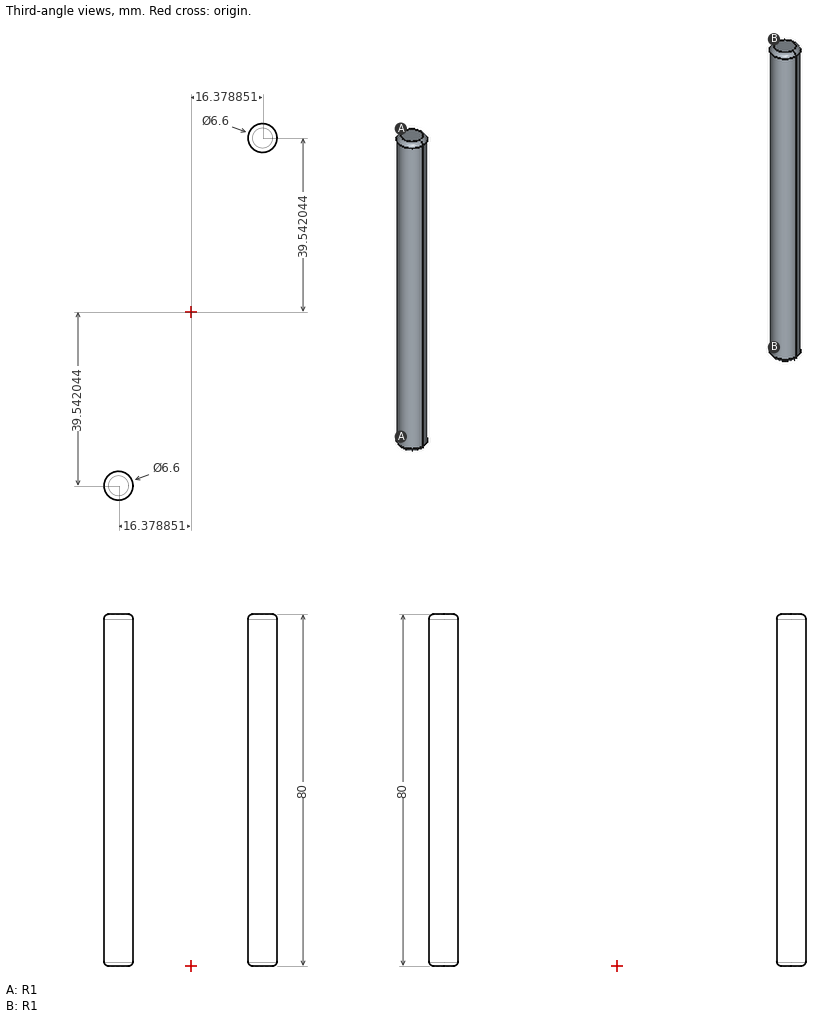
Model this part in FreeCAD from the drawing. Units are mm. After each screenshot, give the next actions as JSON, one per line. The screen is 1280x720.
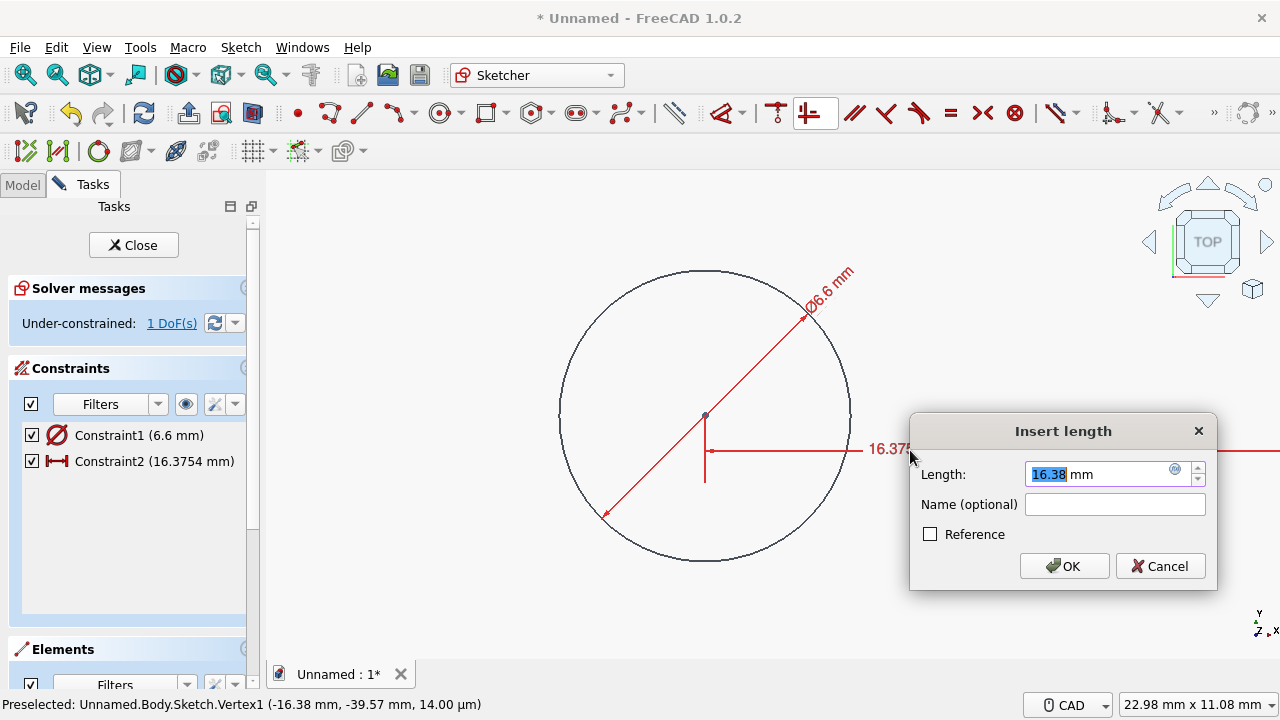
{"action": "type", "text": "16.378851"}
{"action": "key", "text": "Return"}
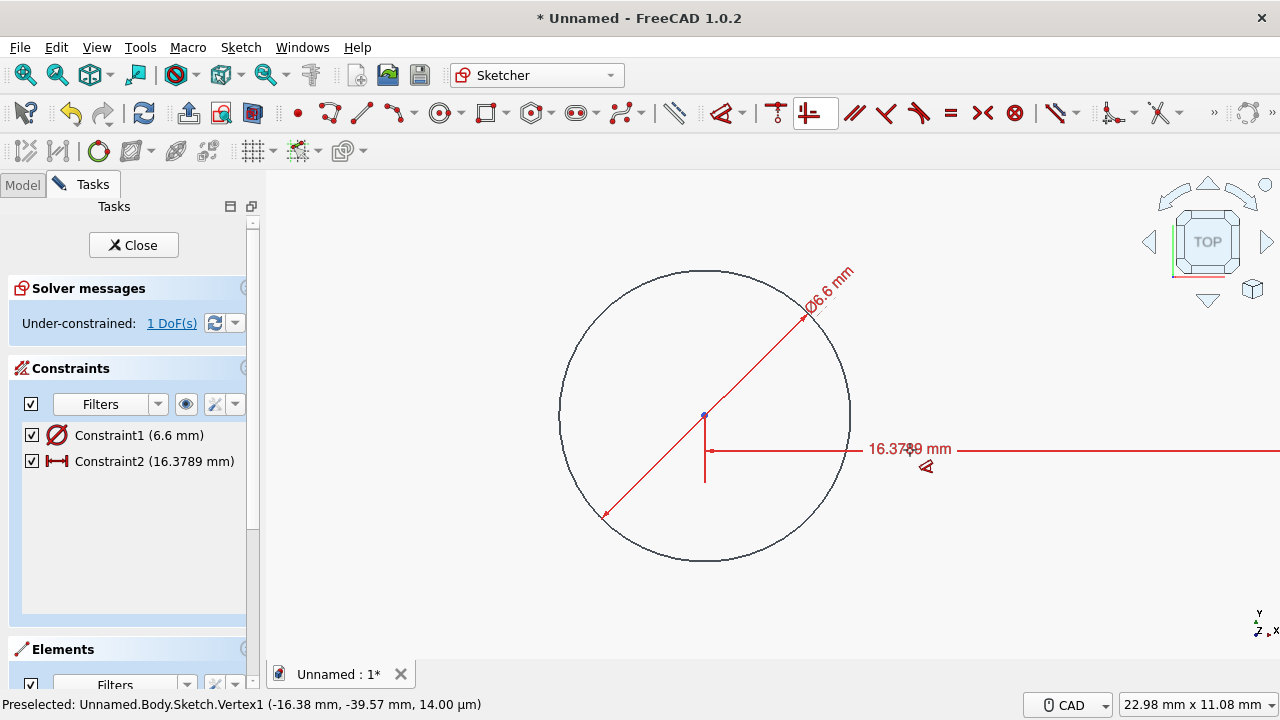
{"action": "left_click", "coordinate": [705, 416]}
{"action": "left_click", "coordinate": [671, 307]}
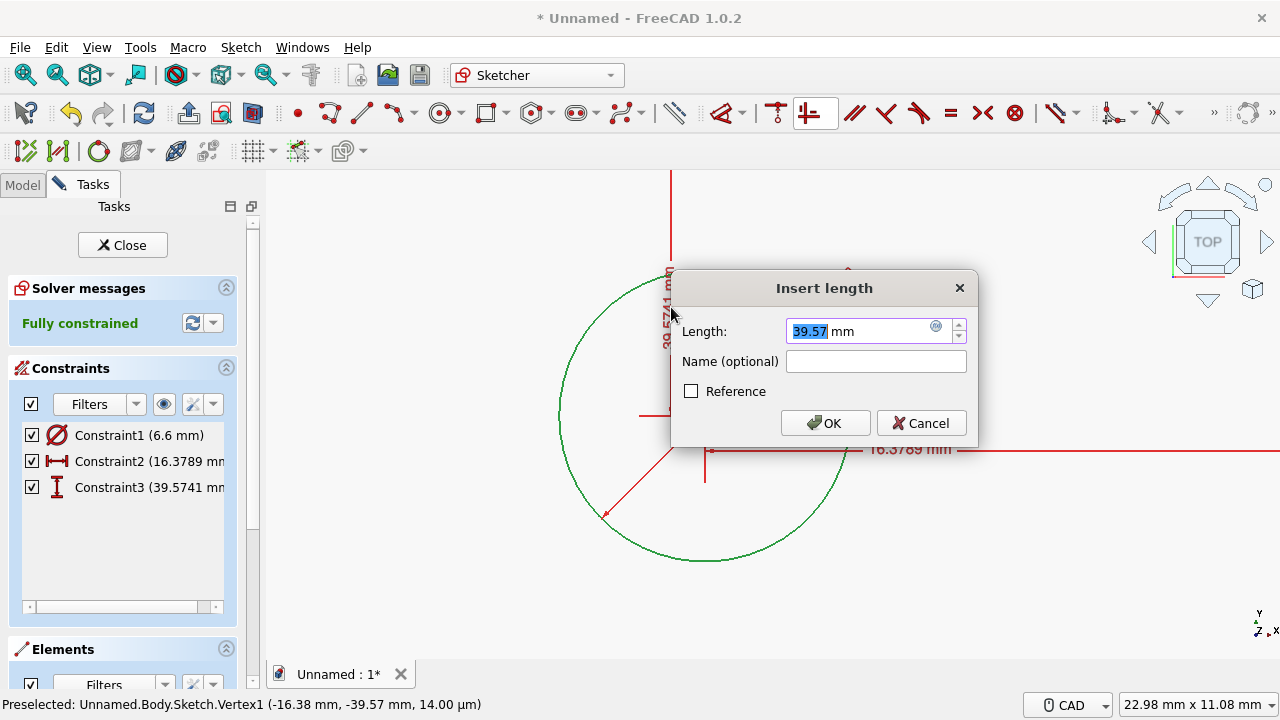
{"action": "type", "text": "39.542044"}
{"action": "key", "text": "Return"}
{"action": "key", "text": "Escape"}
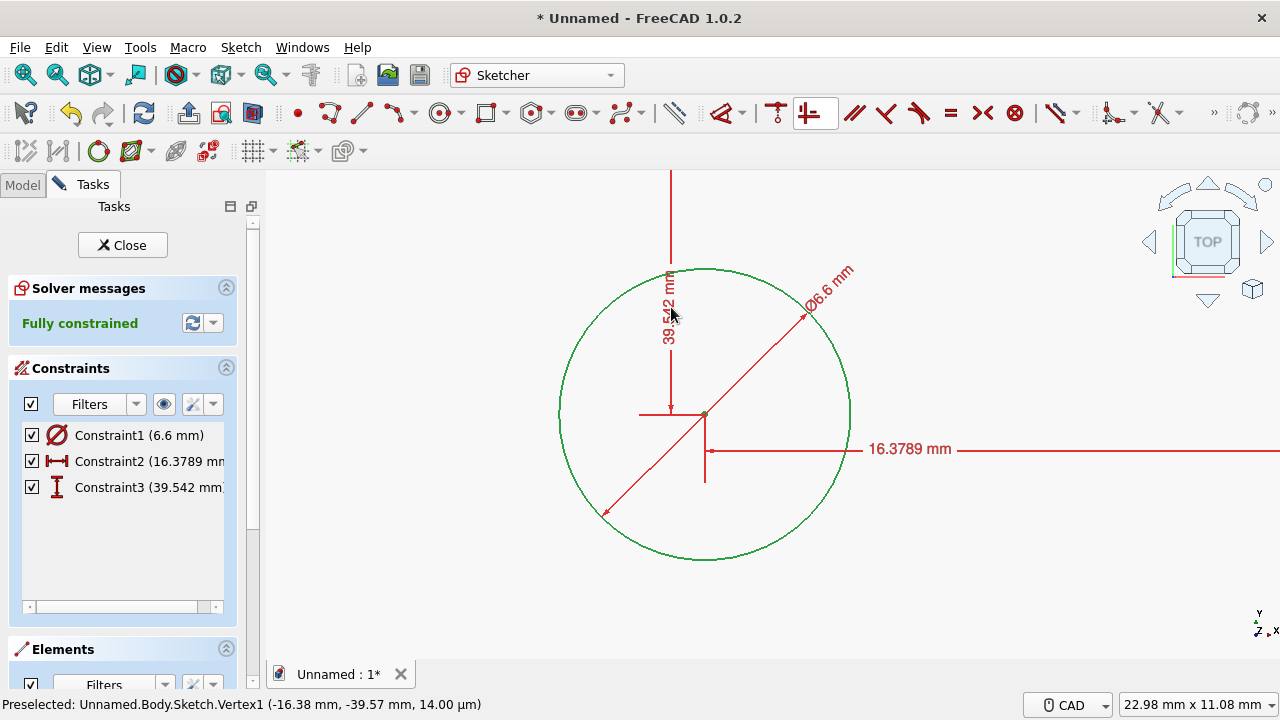
{"action": "left_click", "coordinate": [123, 245]}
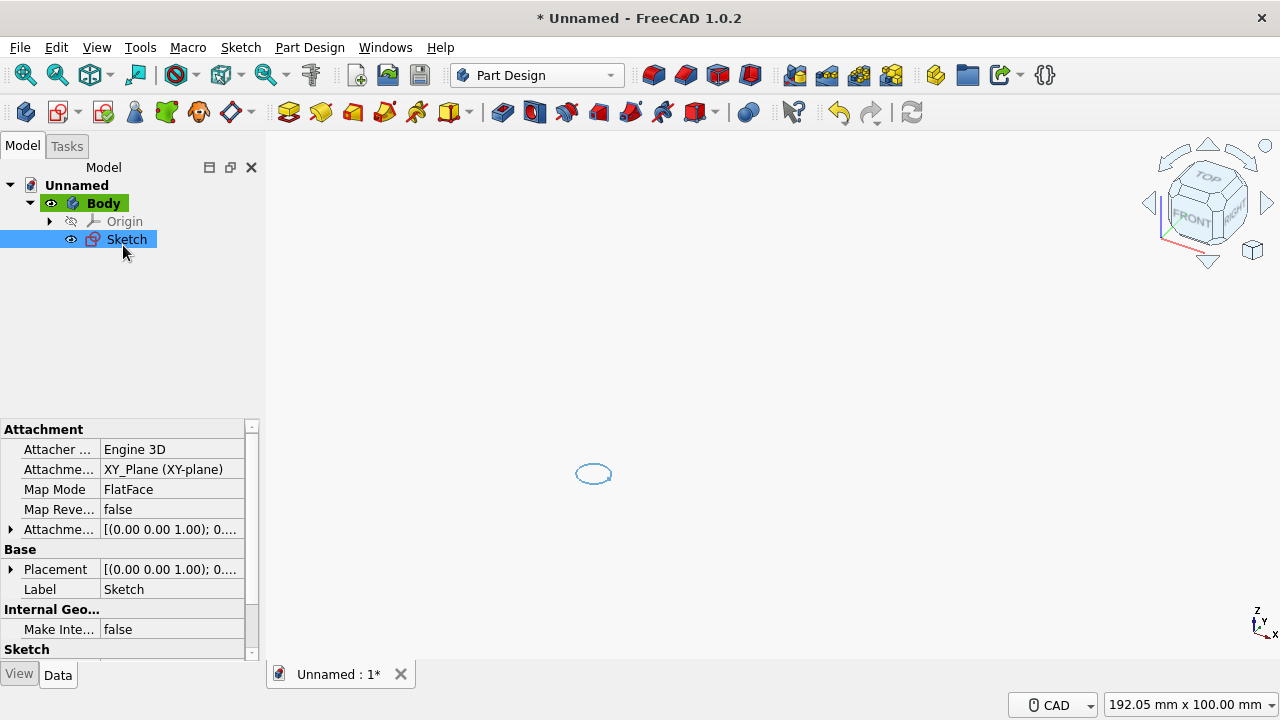
{"action": "left_click", "coordinate": [290, 112]}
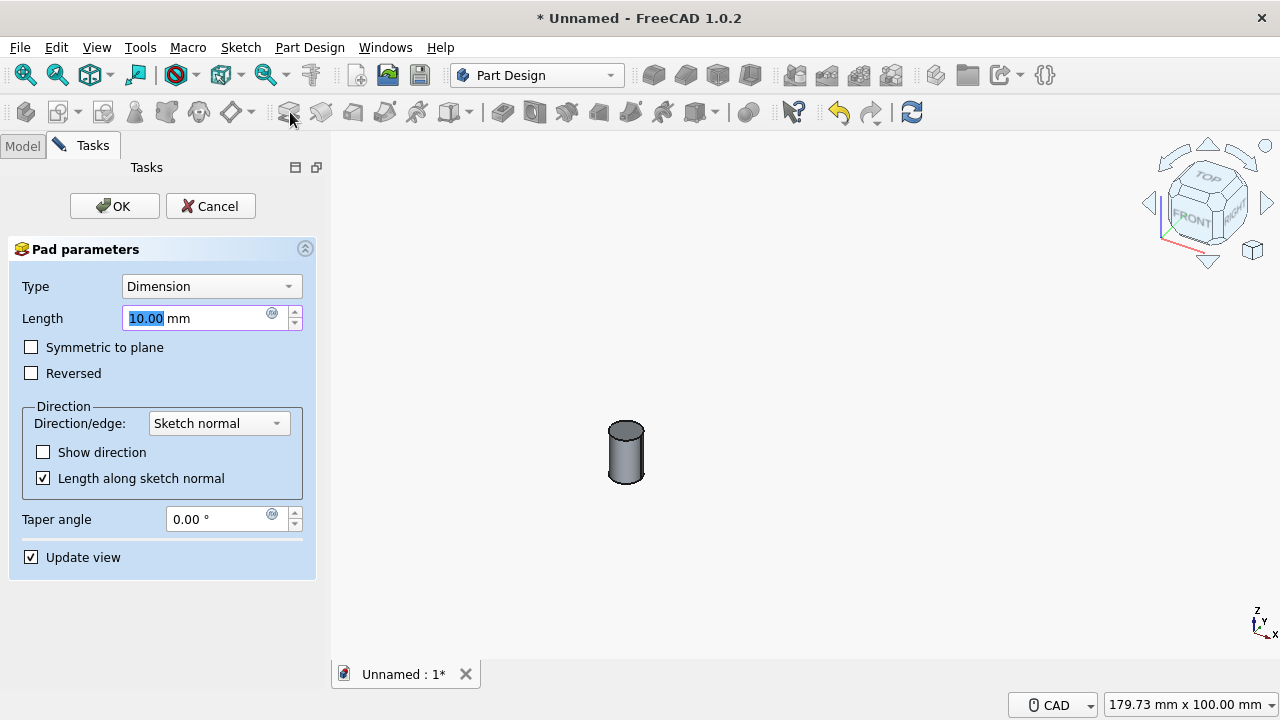
{"action": "type", "text": "80"}
{"action": "key", "text": "Tab"}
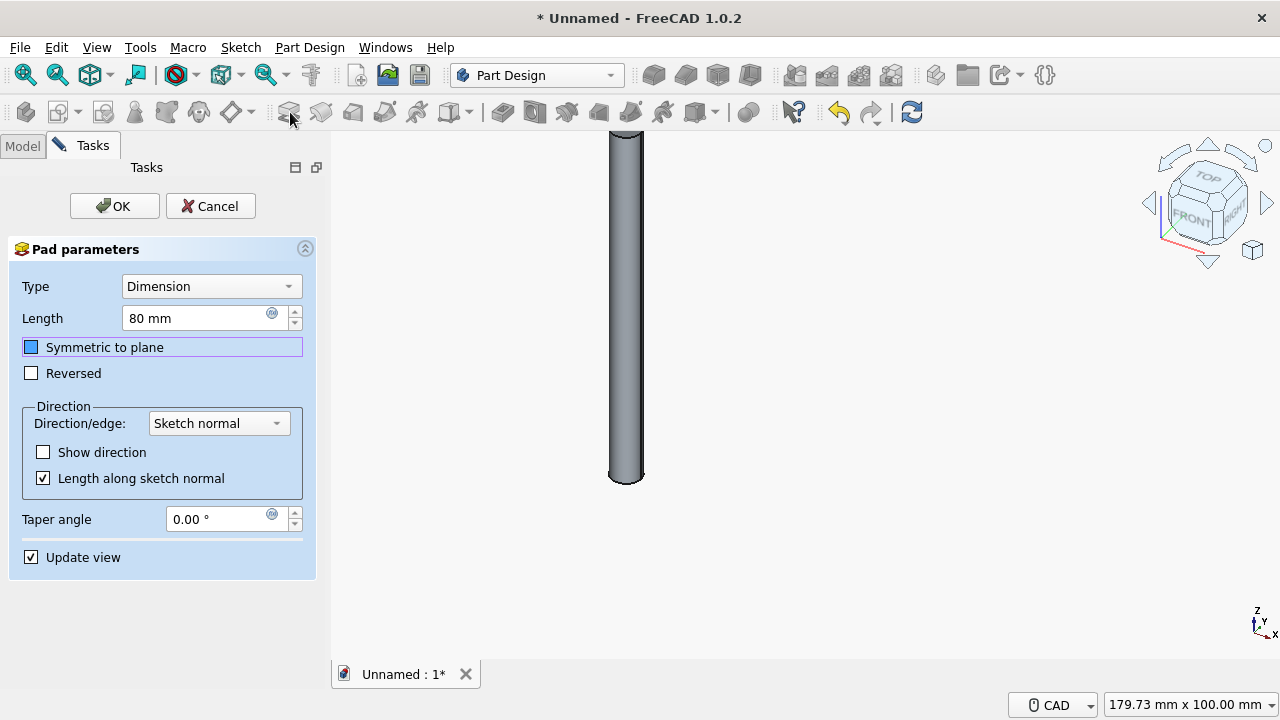
{"action": "left_click", "coordinate": [115, 206]}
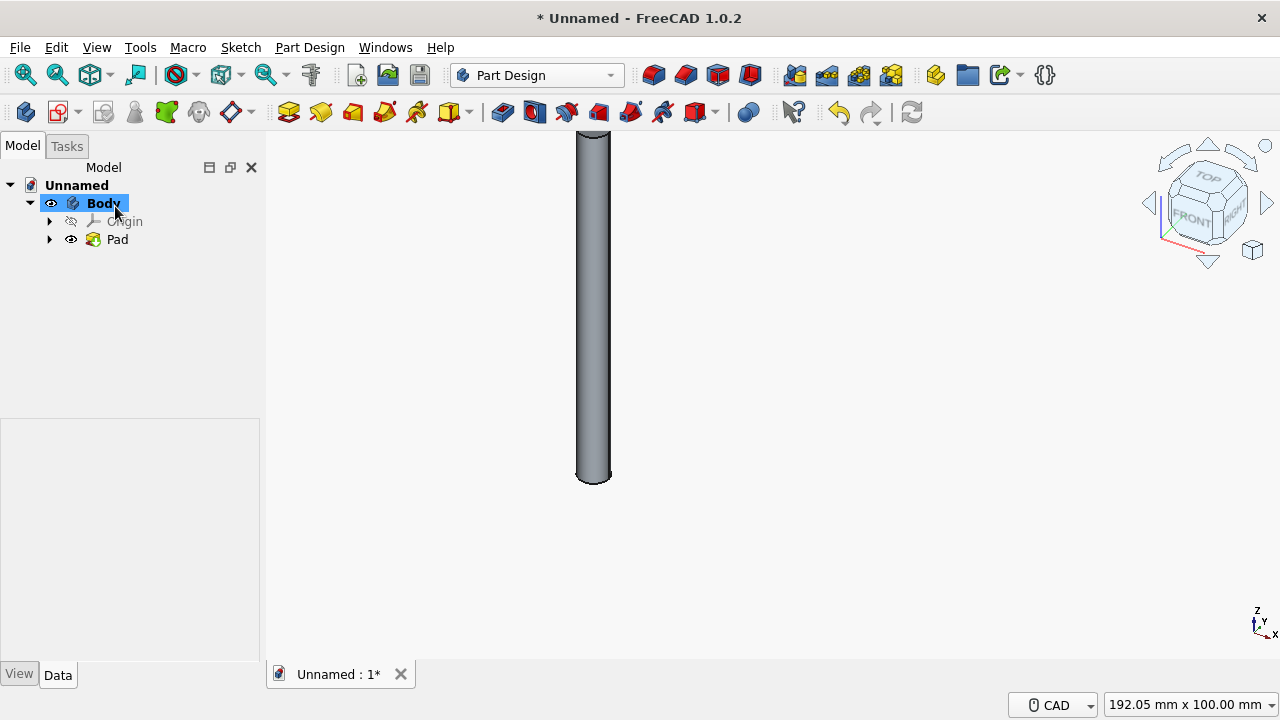
{"action": "left_click", "coordinate": [26, 76]}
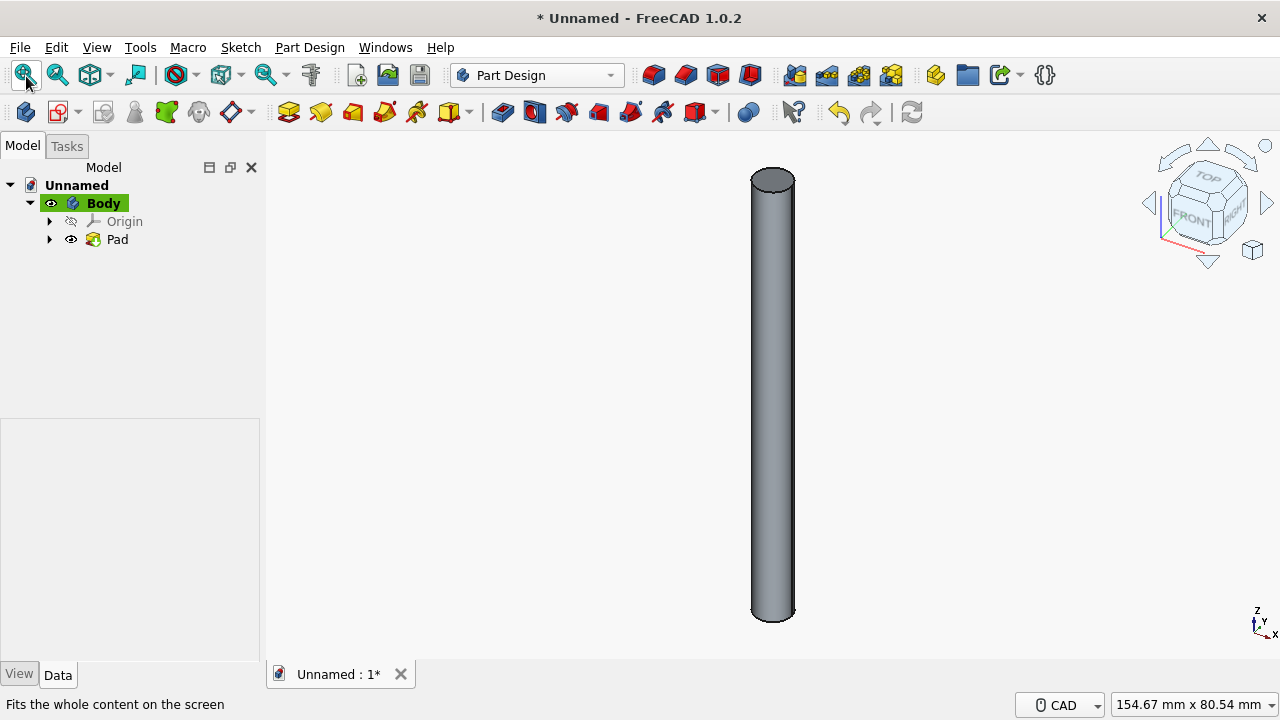
{"action": "left_click", "coordinate": [757, 617]}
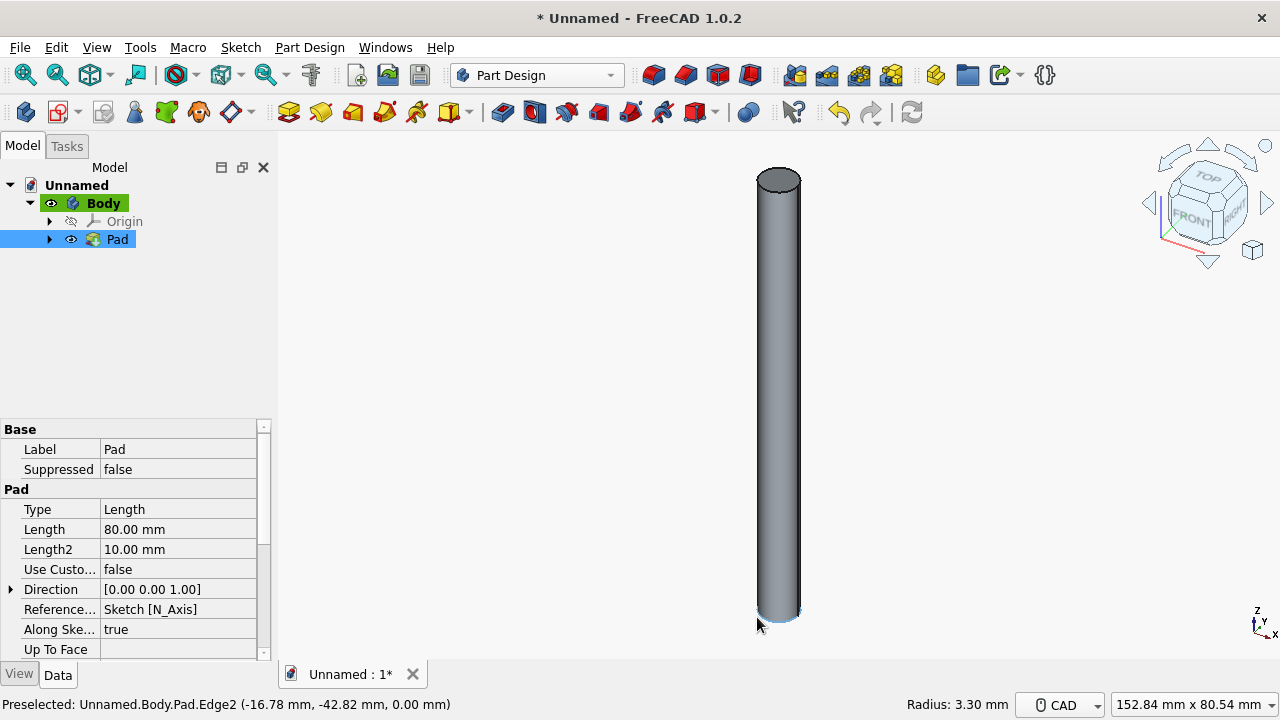
{"action": "left_click", "coordinate": [760, 173], "text": "ctrl"}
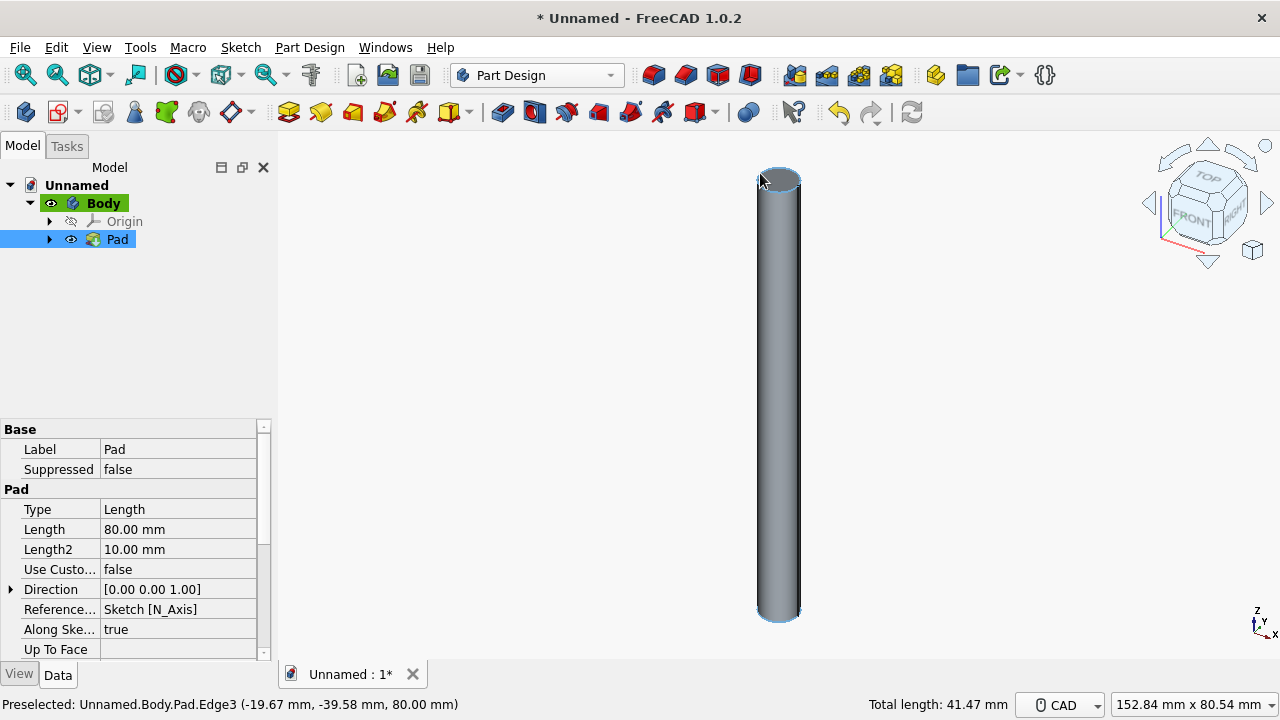
{"action": "left_click", "coordinate": [654, 76]}